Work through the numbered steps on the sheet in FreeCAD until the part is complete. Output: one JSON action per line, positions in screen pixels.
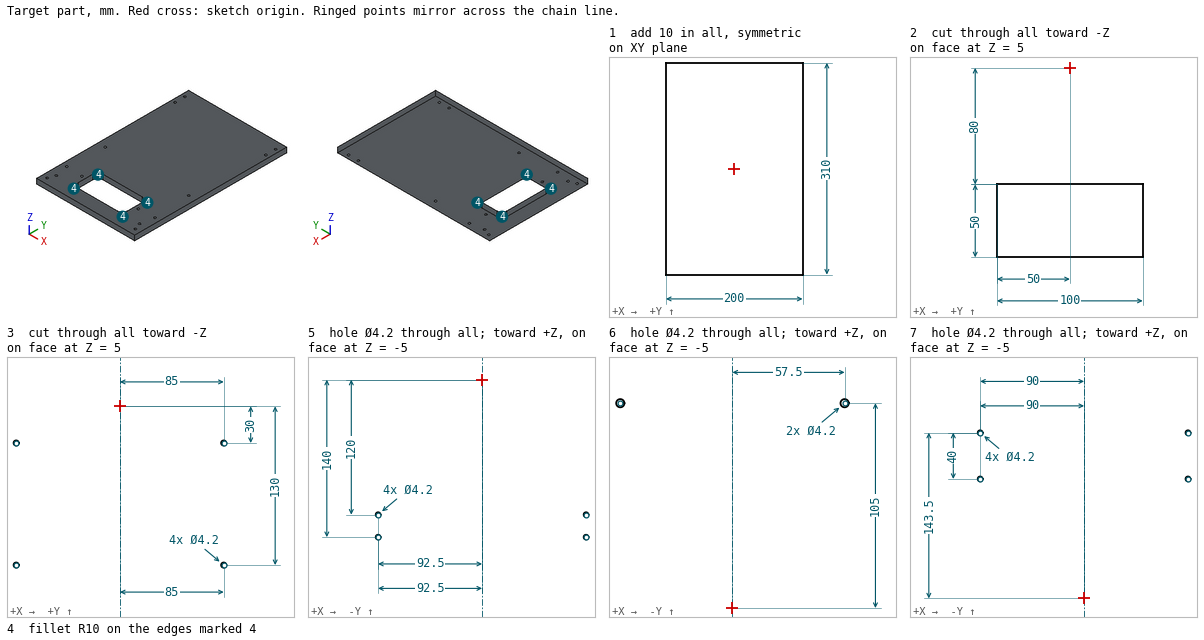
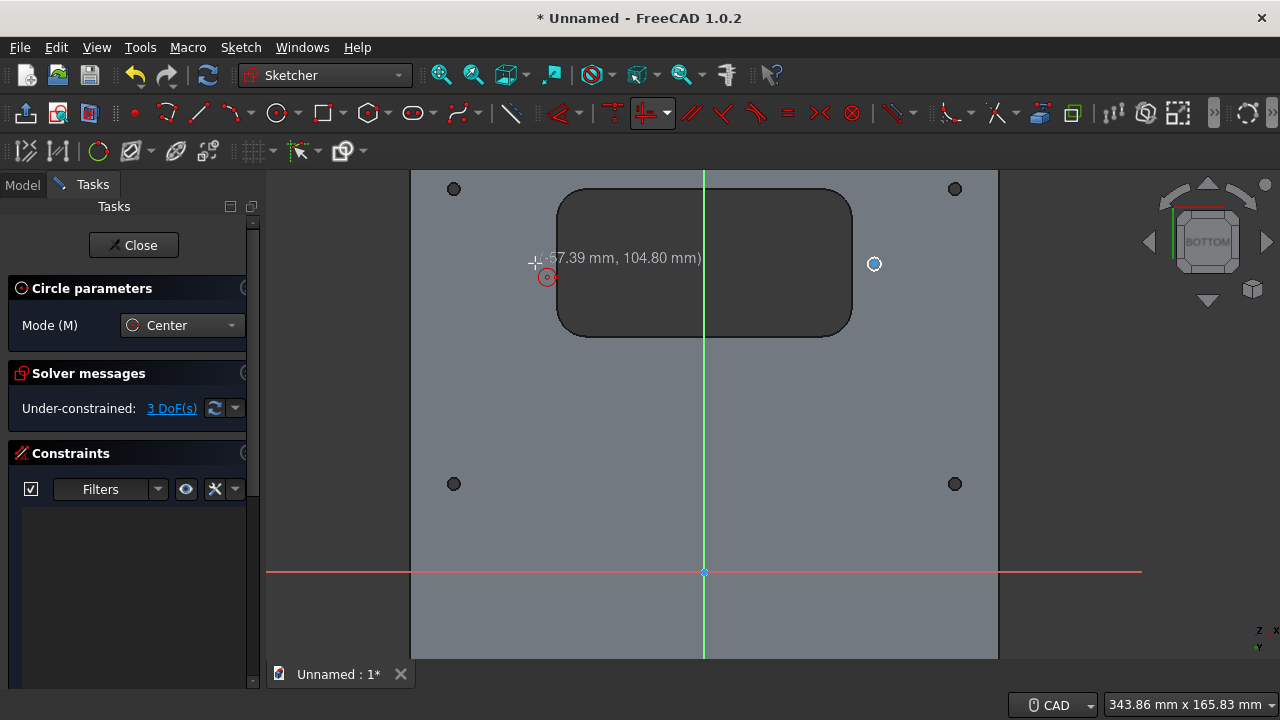
{"action": "left_click", "coordinate": [535, 263]}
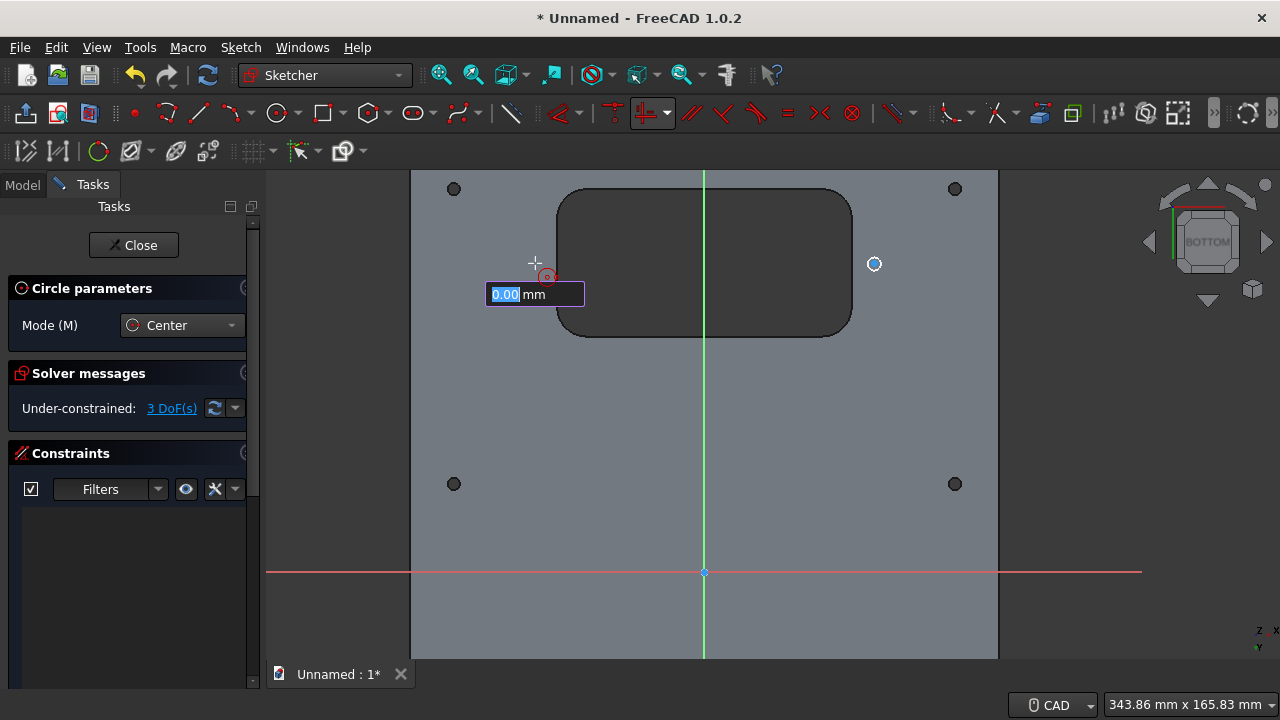
{"action": "scroll", "coordinate": [539, 258], "scroll_direction": "up", "scroll_amount": 5}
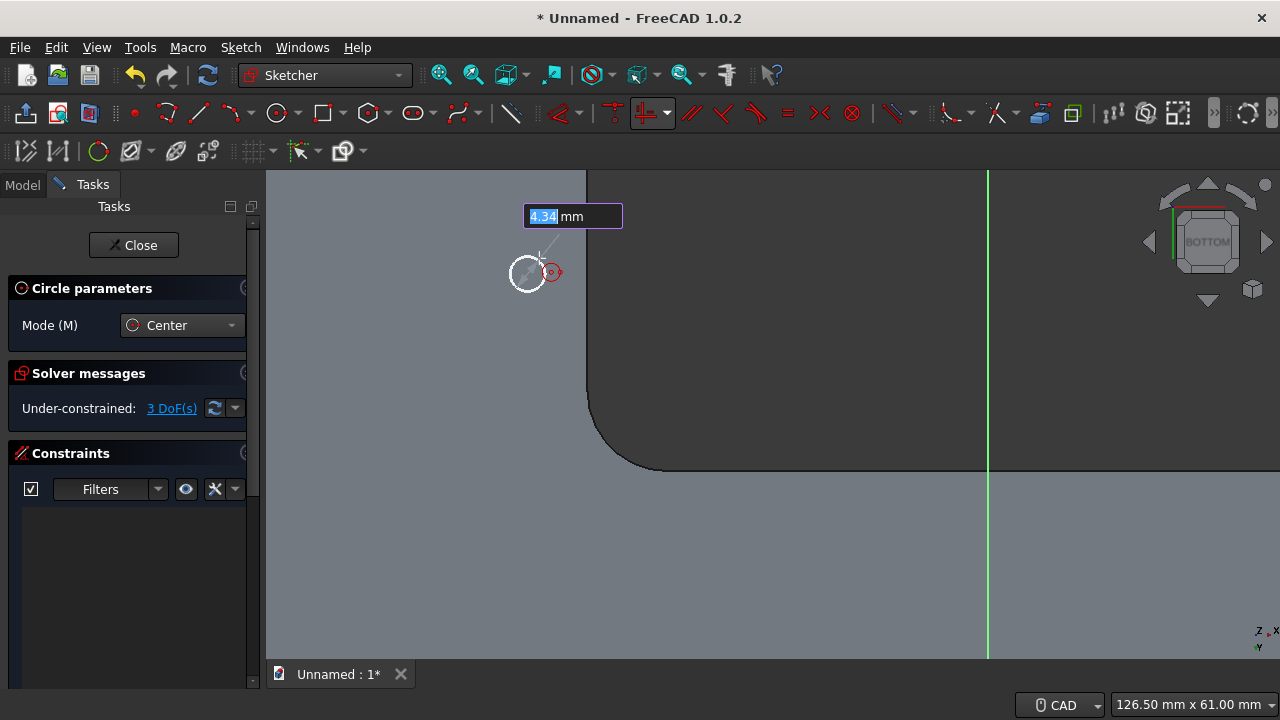
{"action": "left_click", "coordinate": [539, 259]}
{"action": "key", "text": "Escape"}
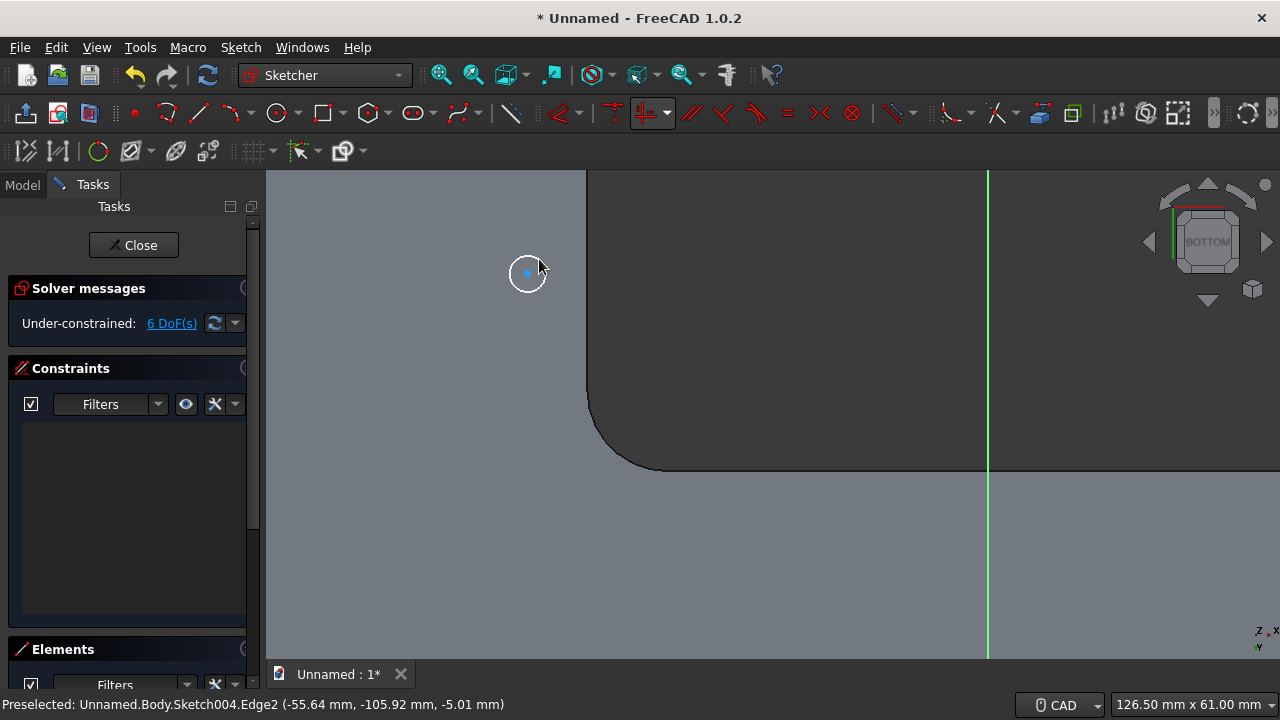
{"action": "scroll", "coordinate": [539, 258], "scroll_direction": "down", "scroll_amount": 5}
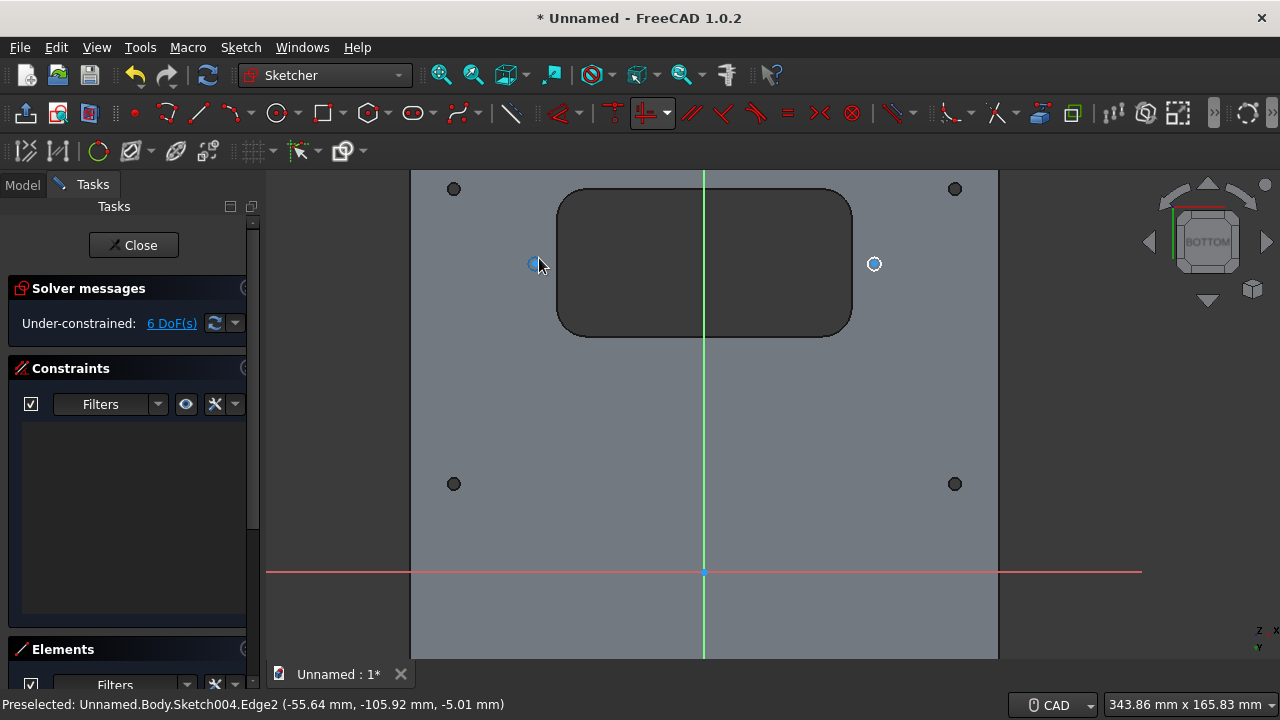
{"action": "scroll", "coordinate": [879, 259], "scroll_direction": "up", "scroll_amount": 4}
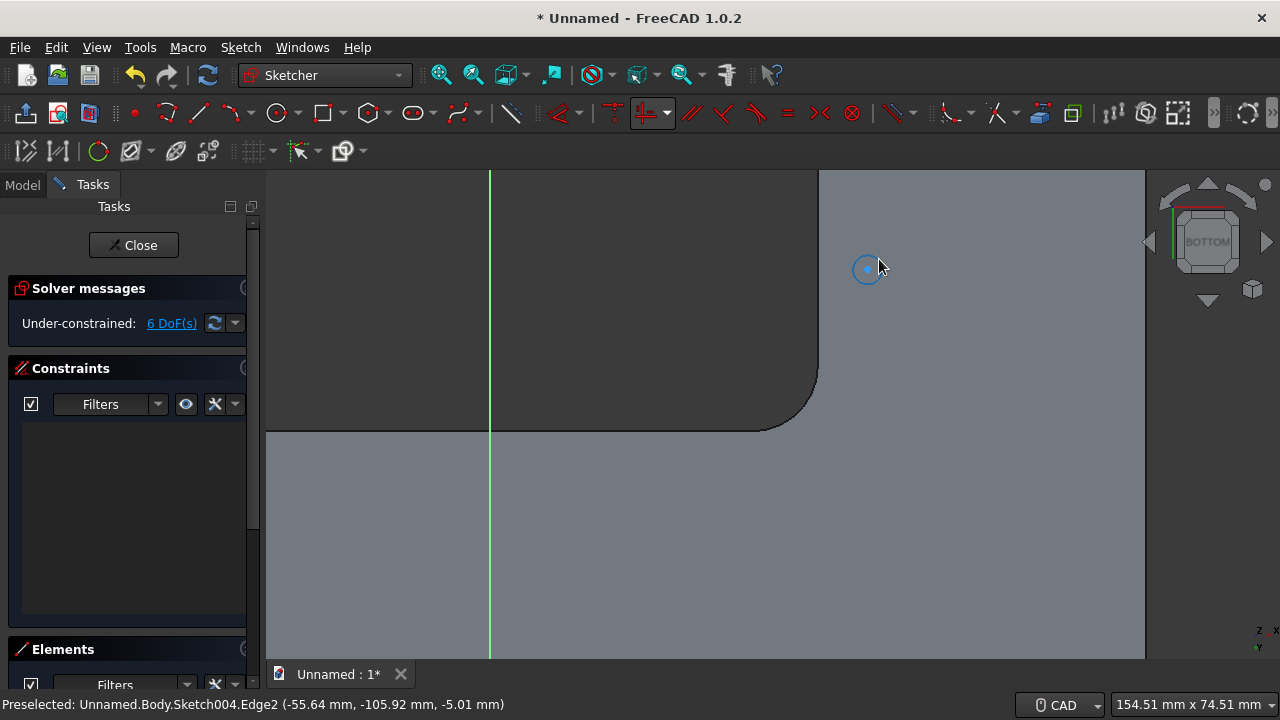
{"action": "left_click", "coordinate": [878, 260]}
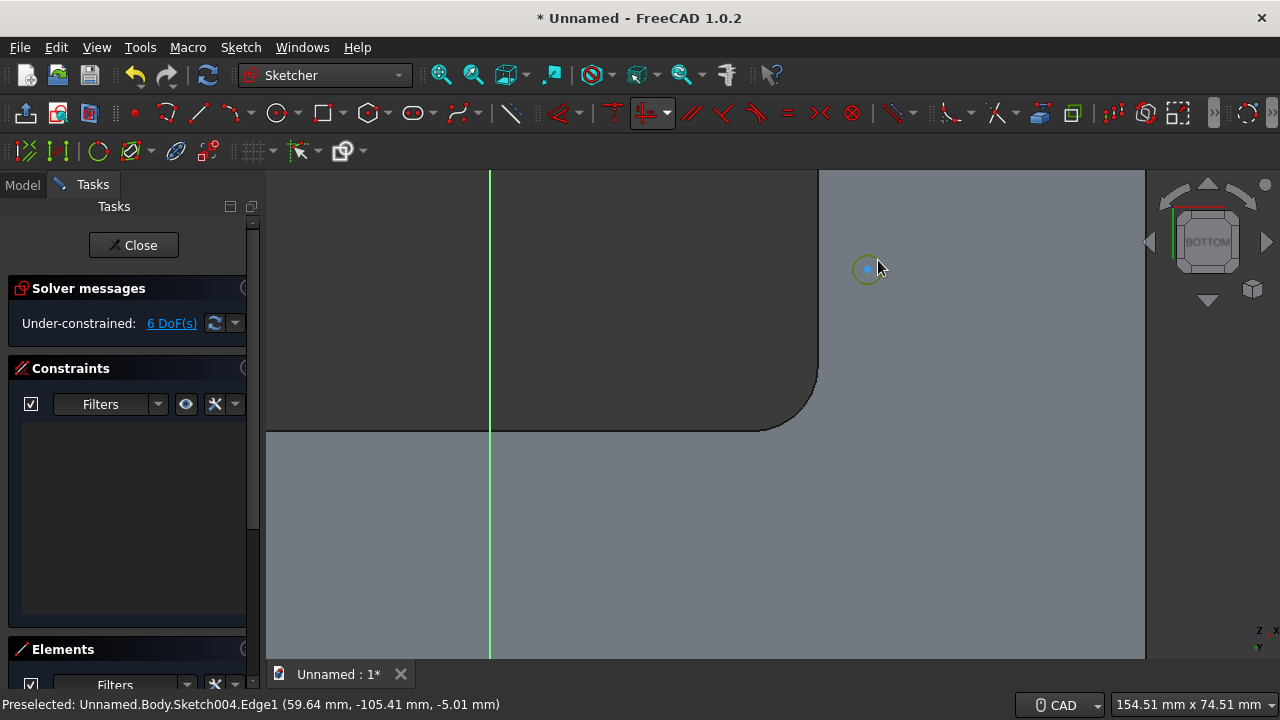
{"action": "scroll", "coordinate": [880, 259], "scroll_direction": "down", "scroll_amount": 4}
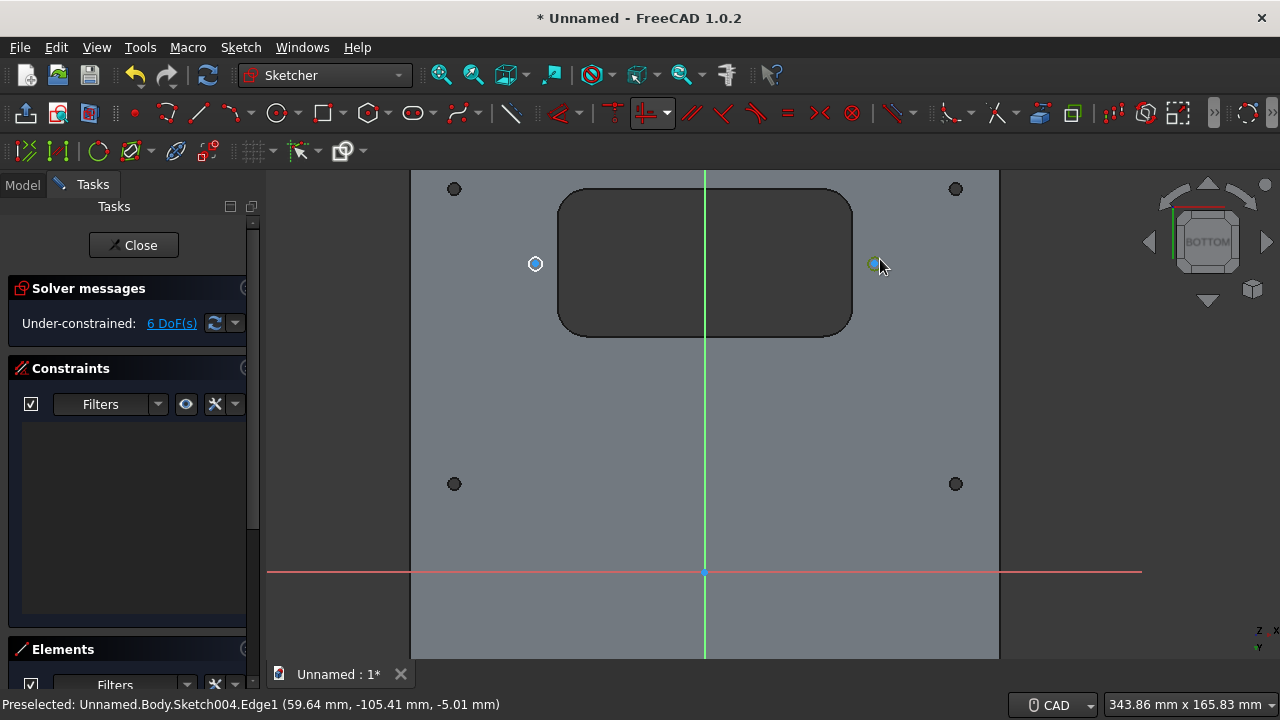
{"action": "scroll", "coordinate": [540, 259], "scroll_direction": "up", "scroll_amount": 4}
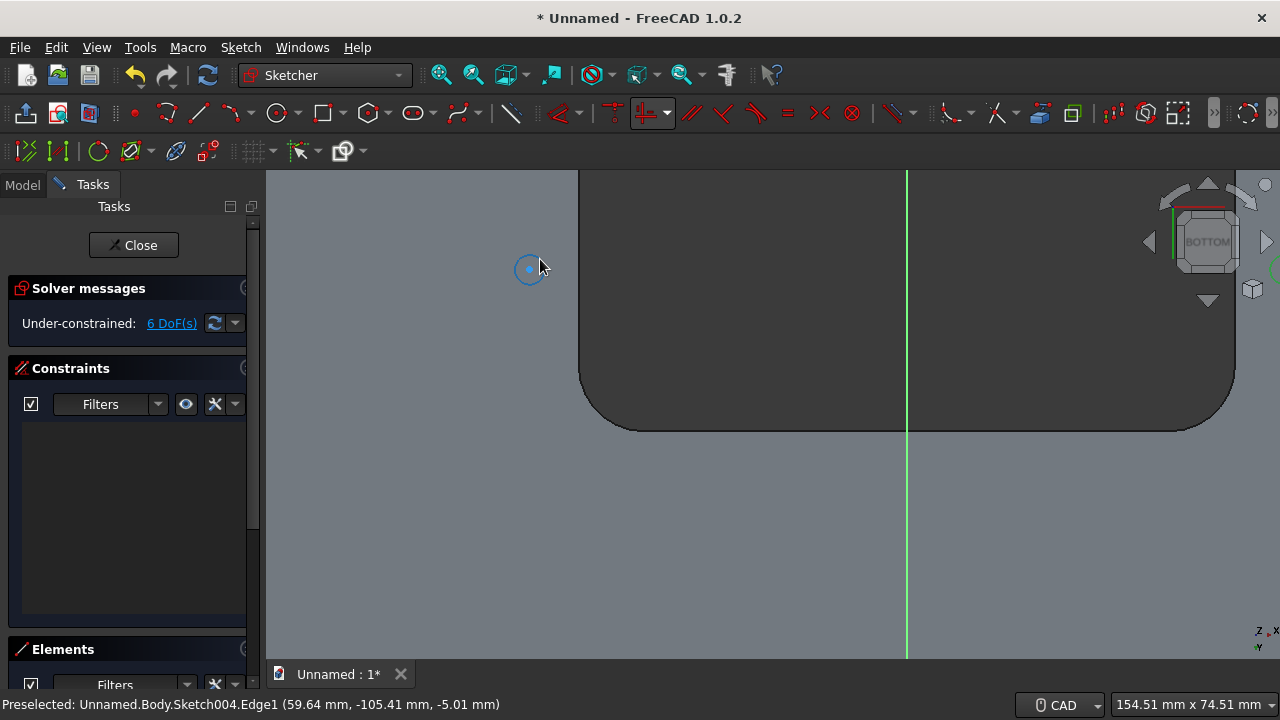
{"action": "left_click", "coordinate": [540, 259]}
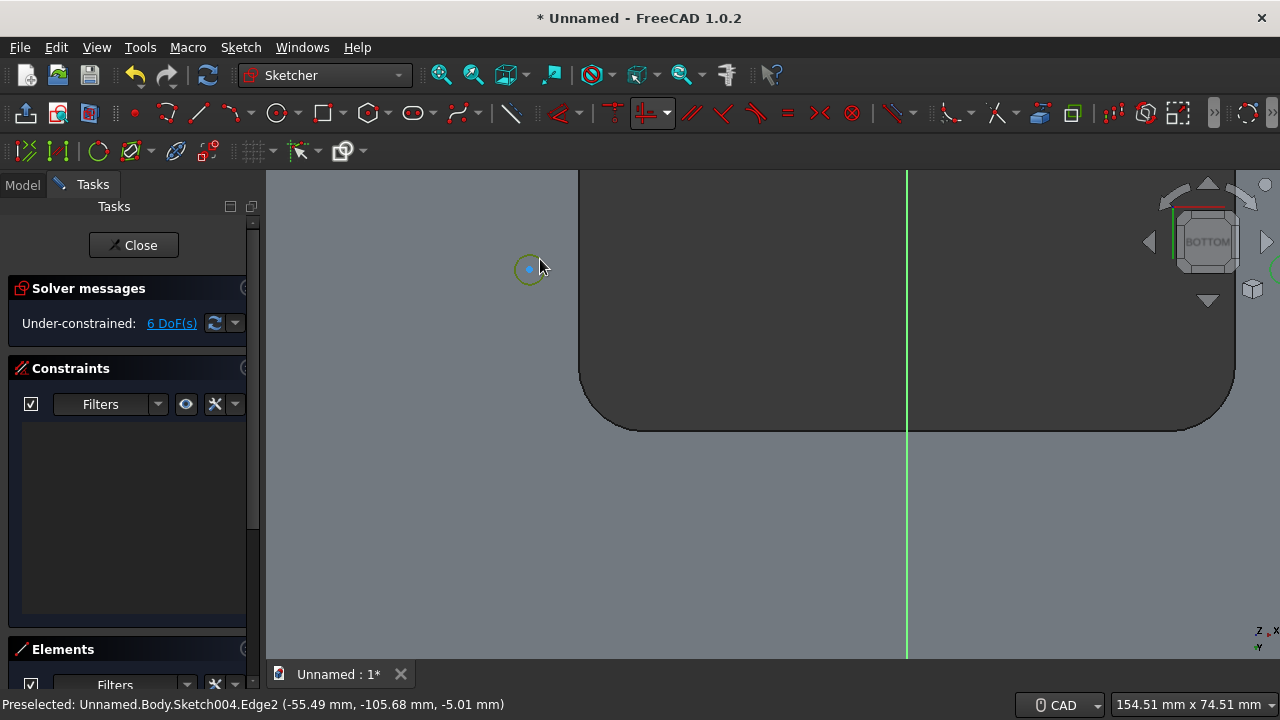
{"action": "left_click", "coordinate": [788, 114]}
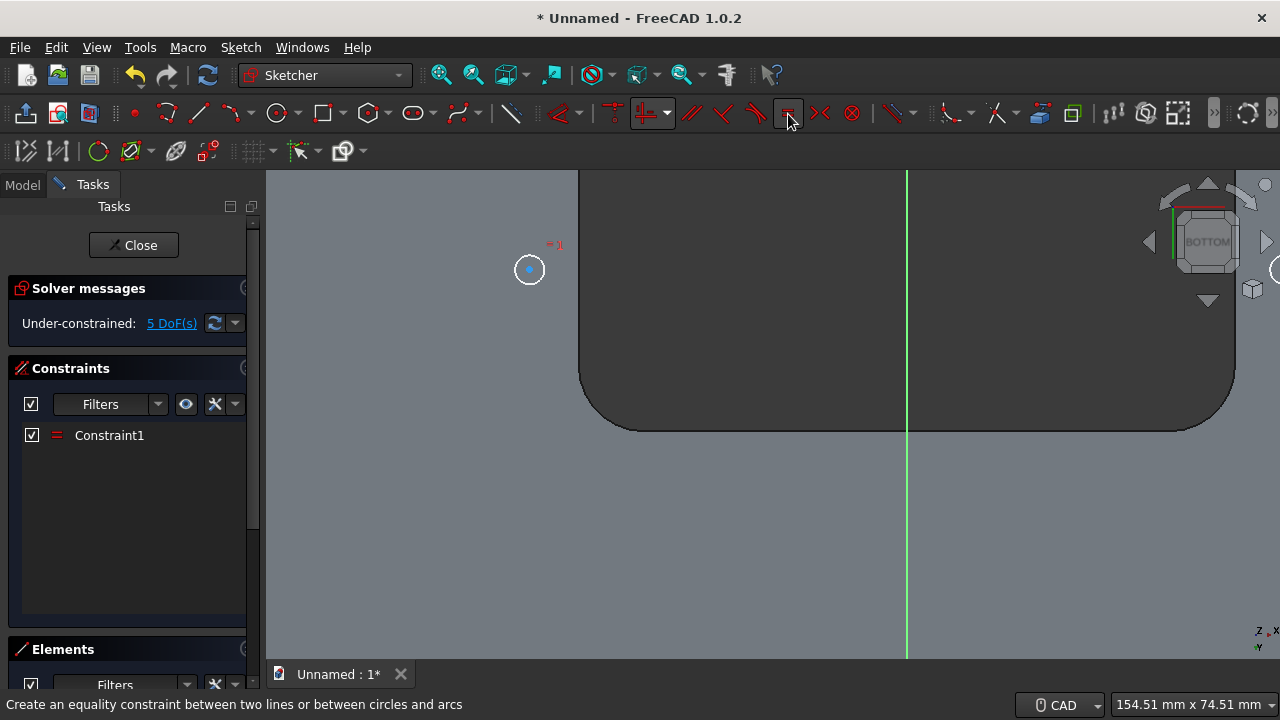
{"action": "scroll", "coordinate": [539, 259], "scroll_direction": "down", "scroll_amount": 4}